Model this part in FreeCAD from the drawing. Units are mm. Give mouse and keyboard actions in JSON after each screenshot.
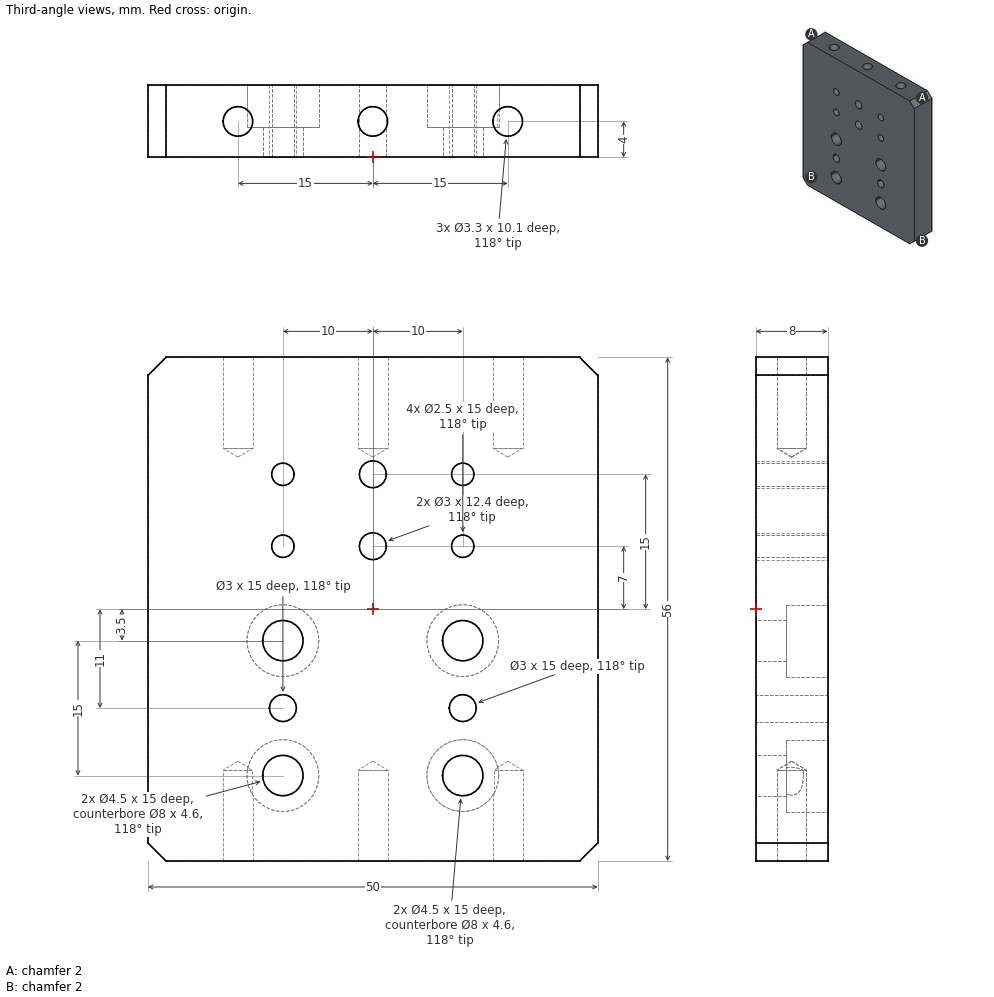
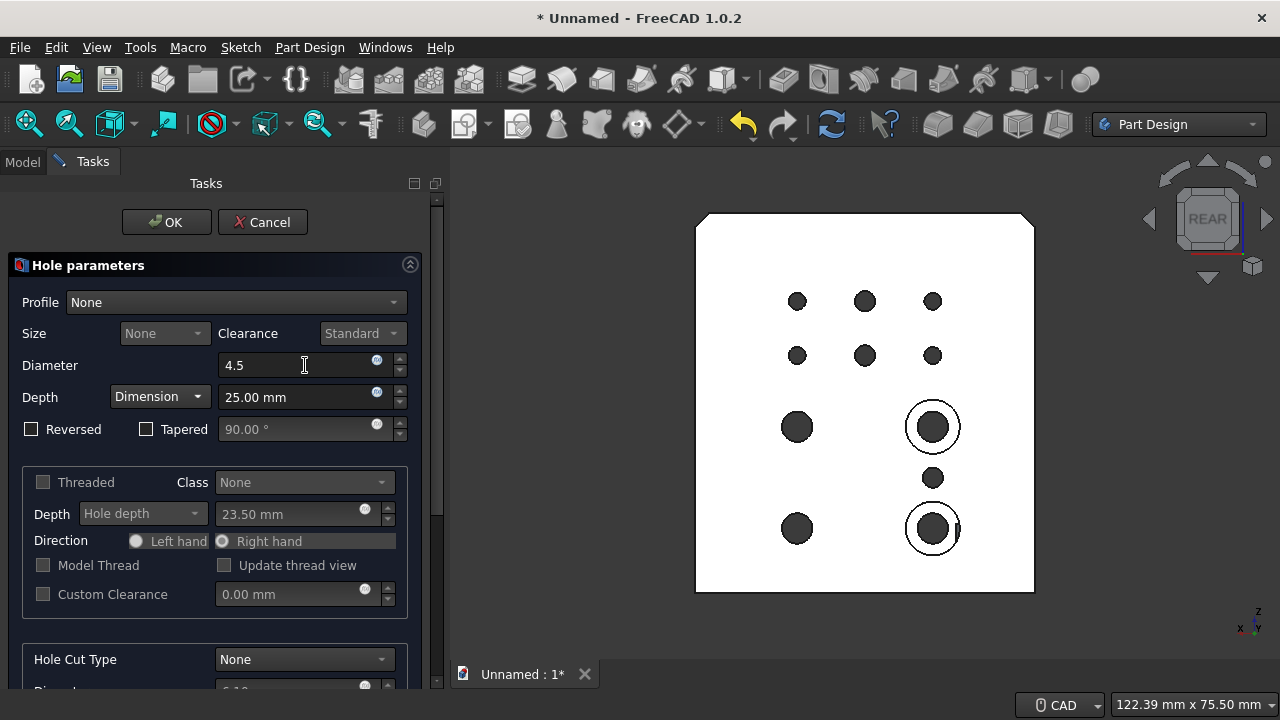
{"action": "triple_click", "coordinate": [305, 397]}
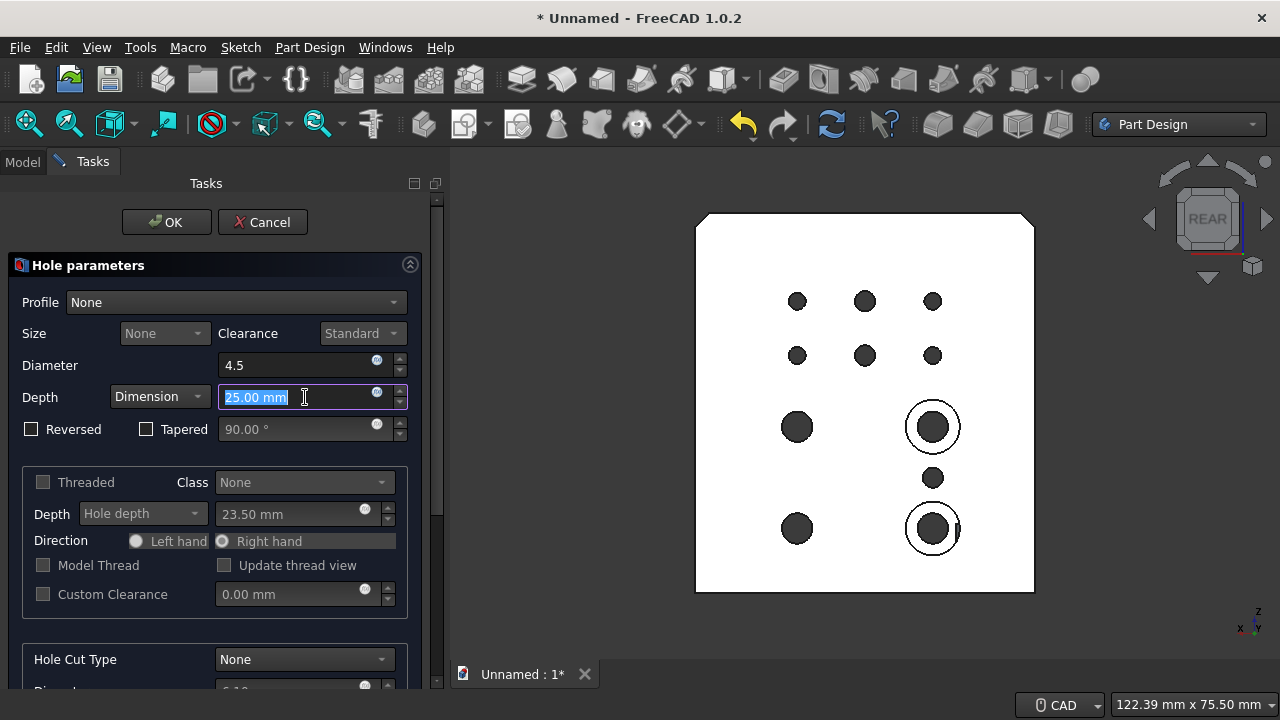
{"action": "type", "text": "15"}
{"action": "key", "text": "Tab"}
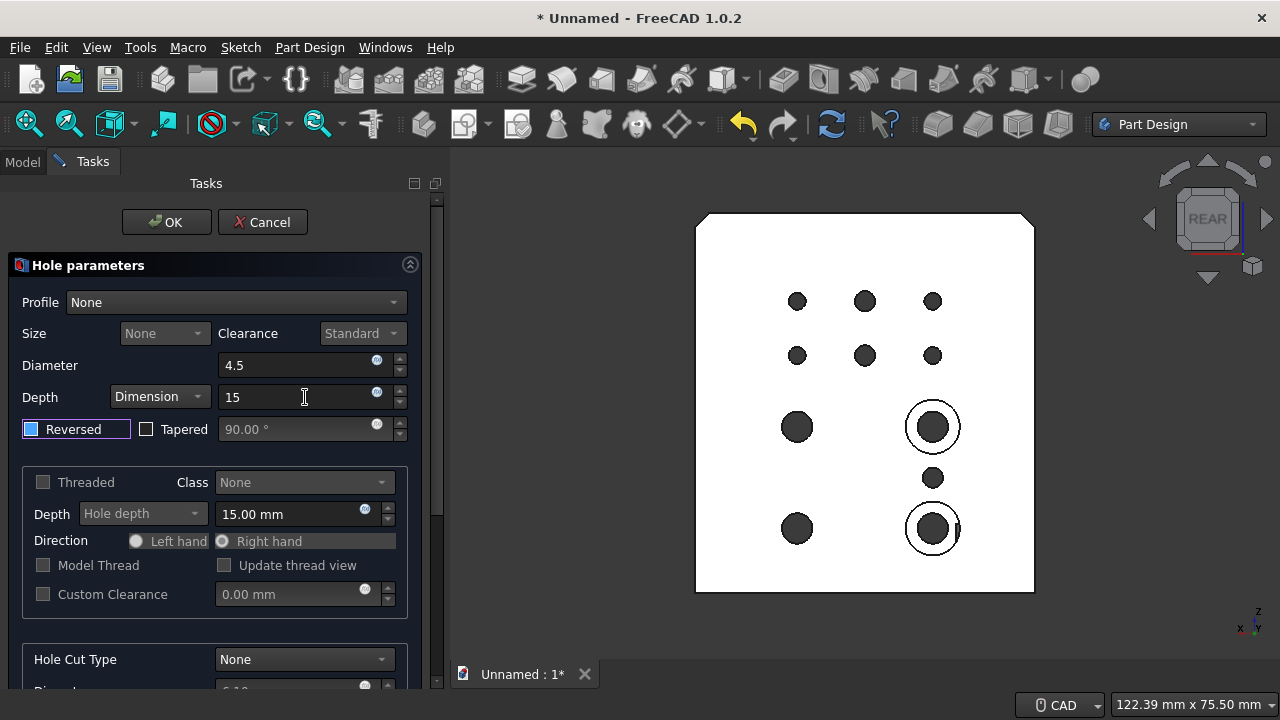
{"action": "left_click", "coordinate": [306, 660]}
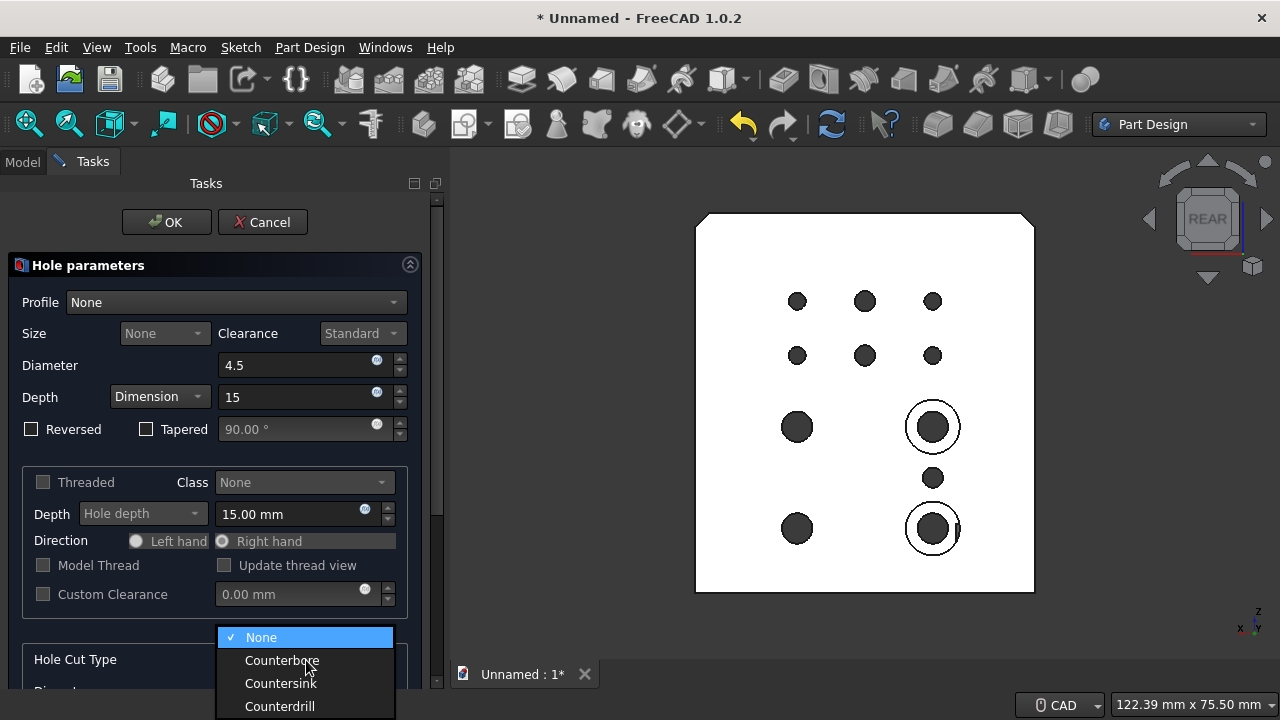
{"action": "left_click", "coordinate": [304, 660]}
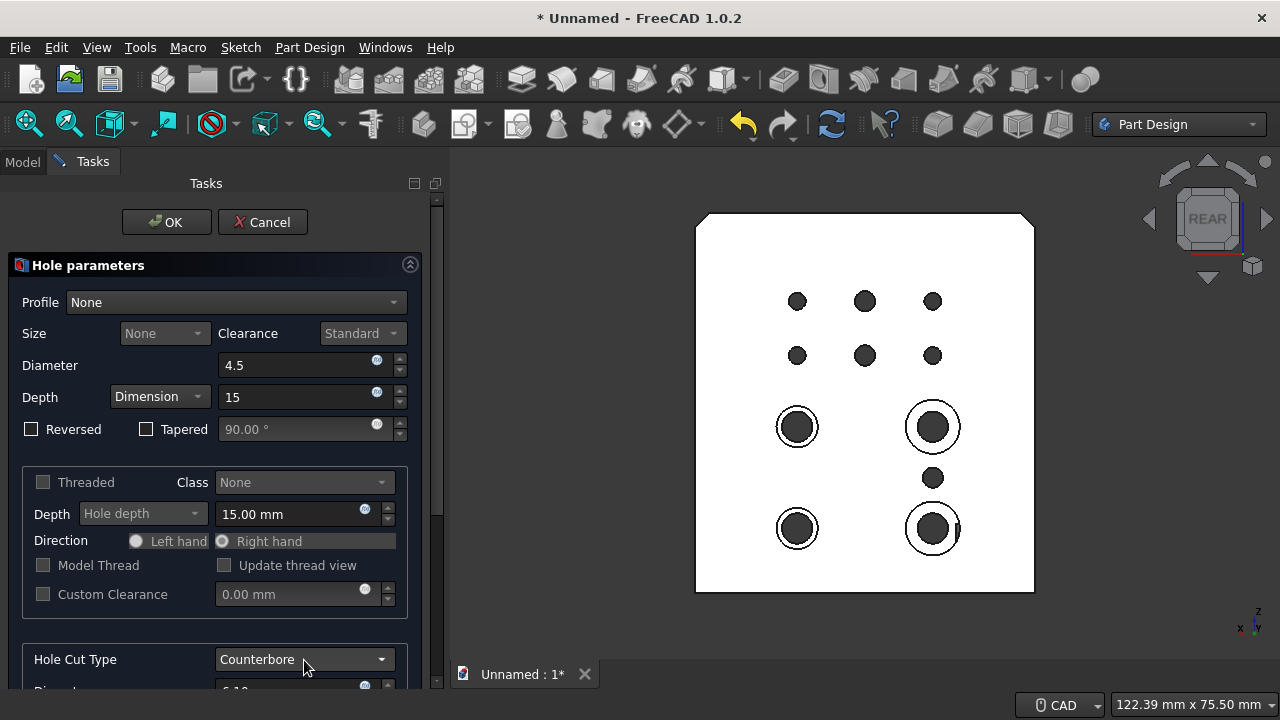
{"action": "scroll", "coordinate": [437, 440], "scroll_direction": "down", "scroll_amount": 2}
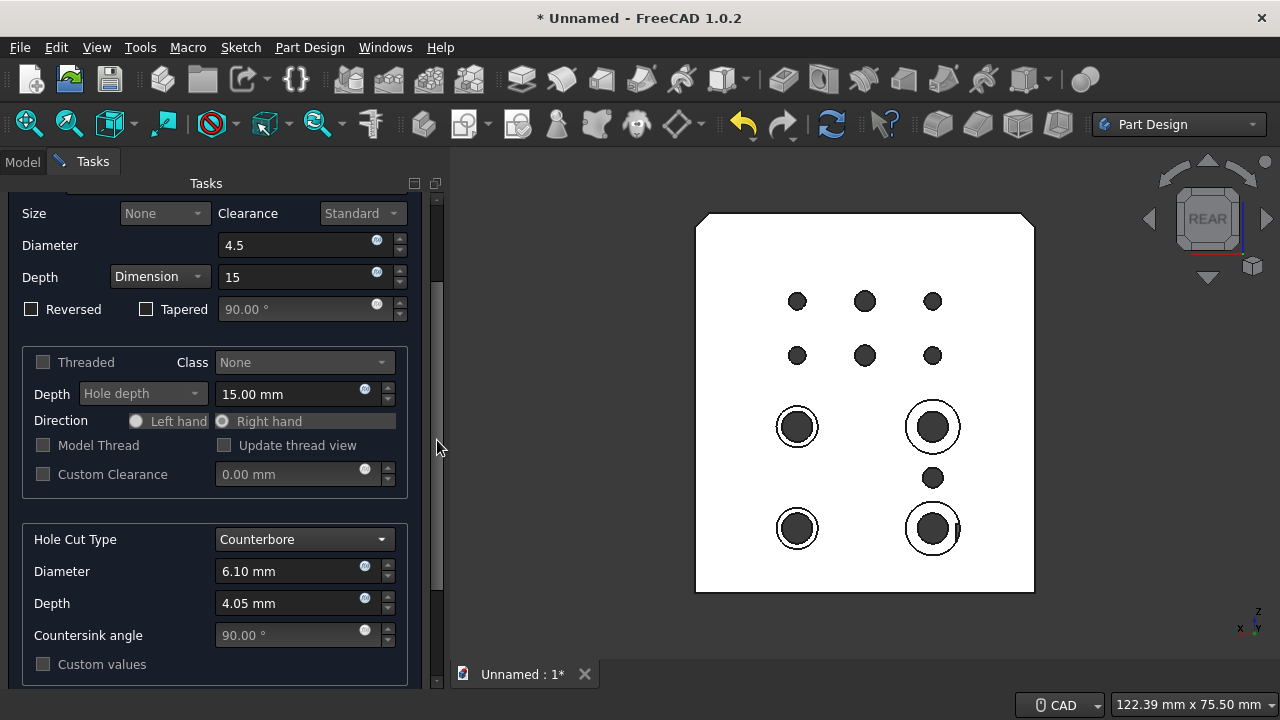
{"action": "triple_click", "coordinate": [298, 571]}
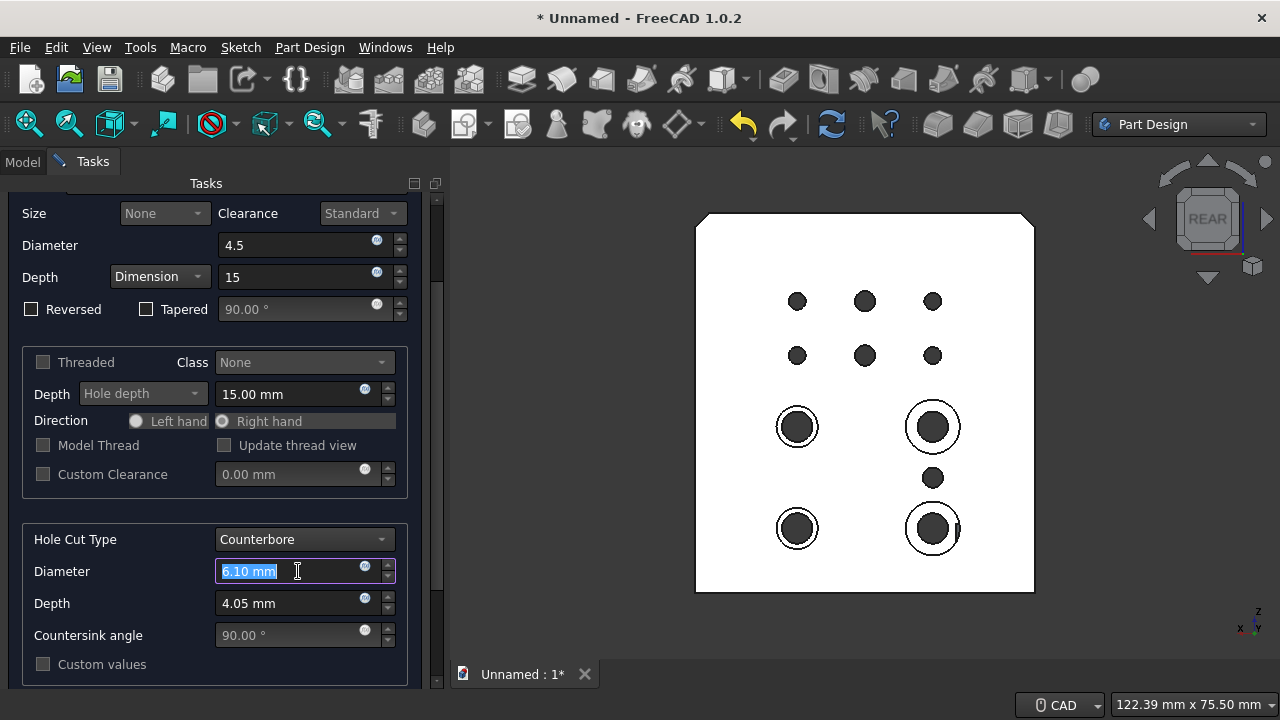
{"action": "type", "text": "8"}
{"action": "key", "text": "Tab"}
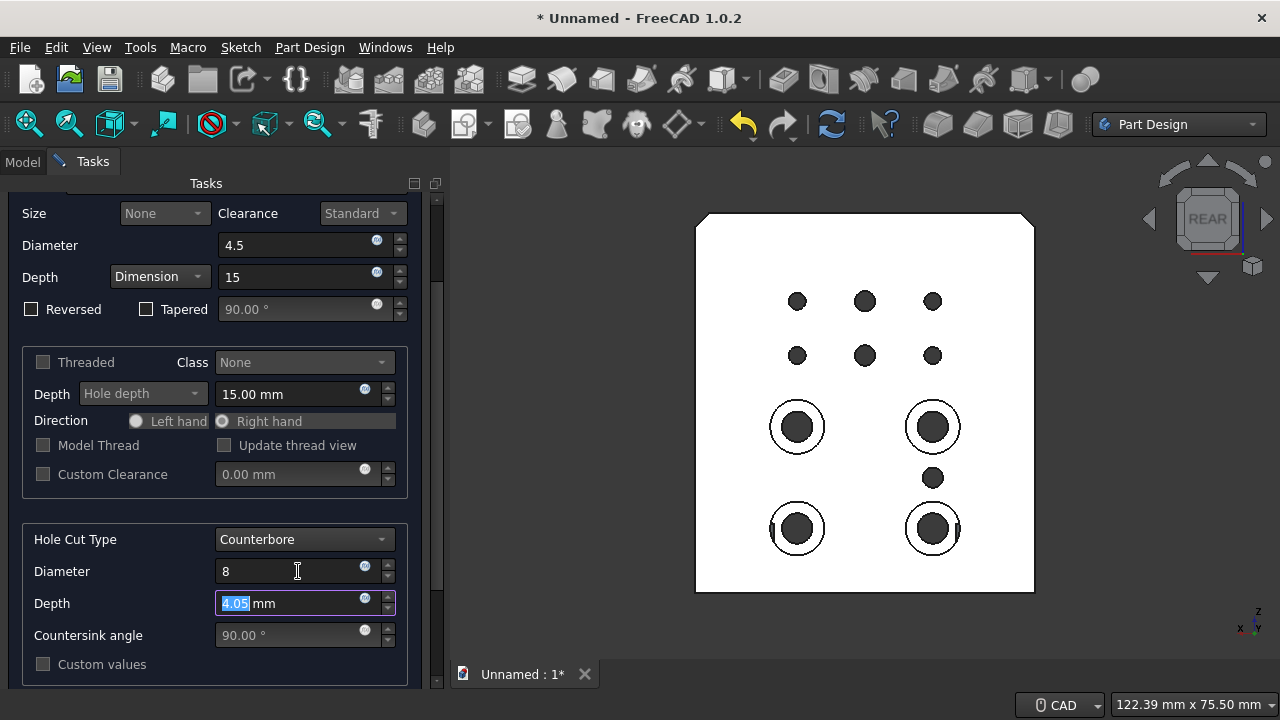
{"action": "type", "text": "4.6"}
{"action": "key", "text": "Tab"}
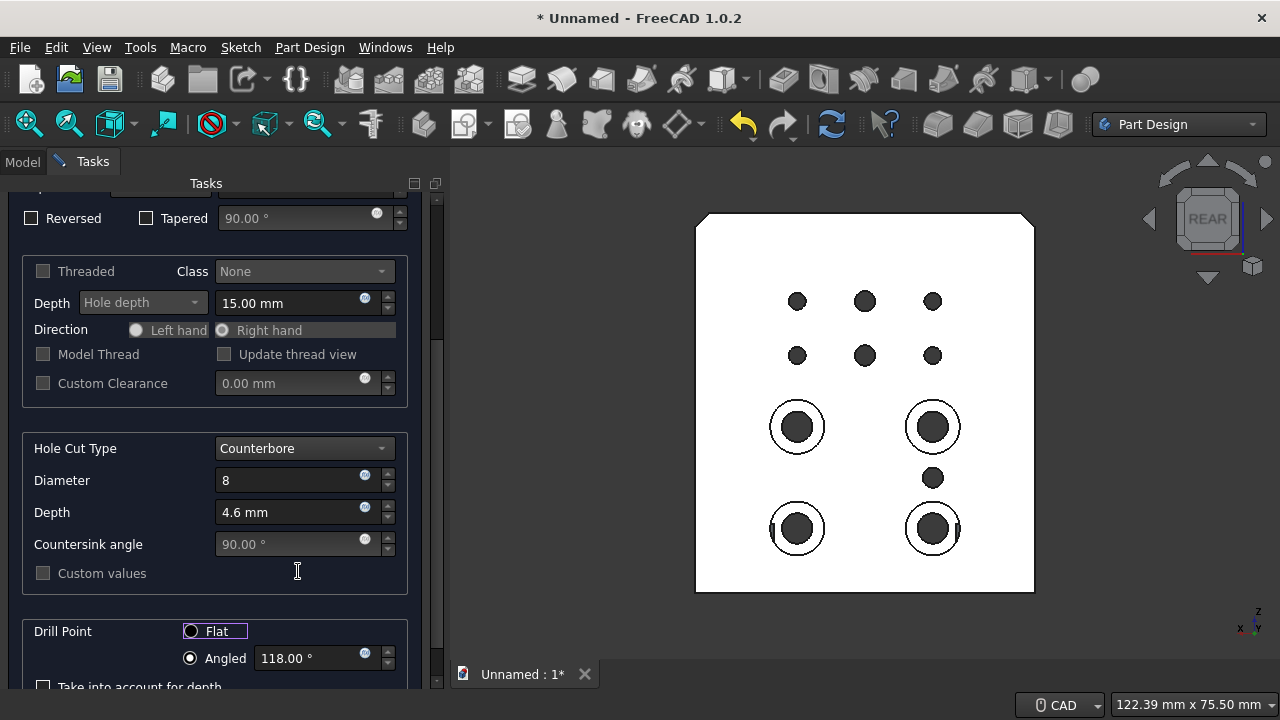
{"action": "scroll", "coordinate": [437, 440], "scroll_direction": "up", "scroll_amount": 5}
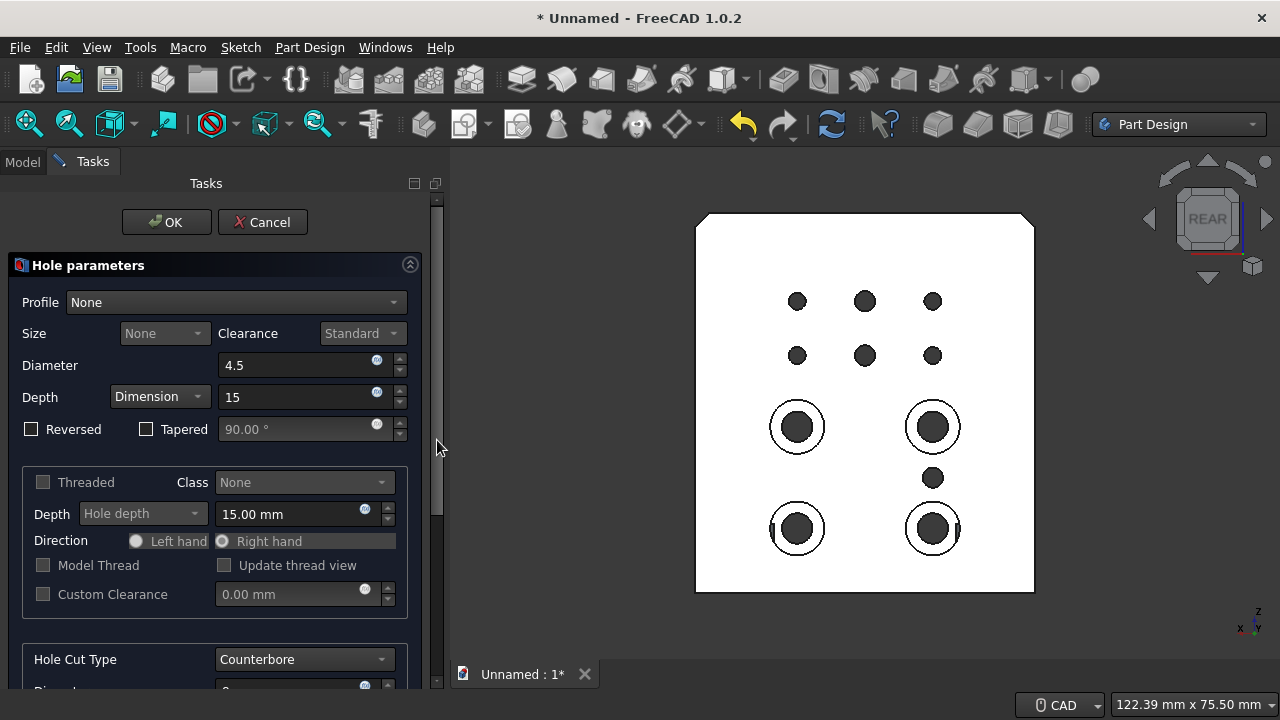
{"action": "left_click", "coordinate": [167, 222]}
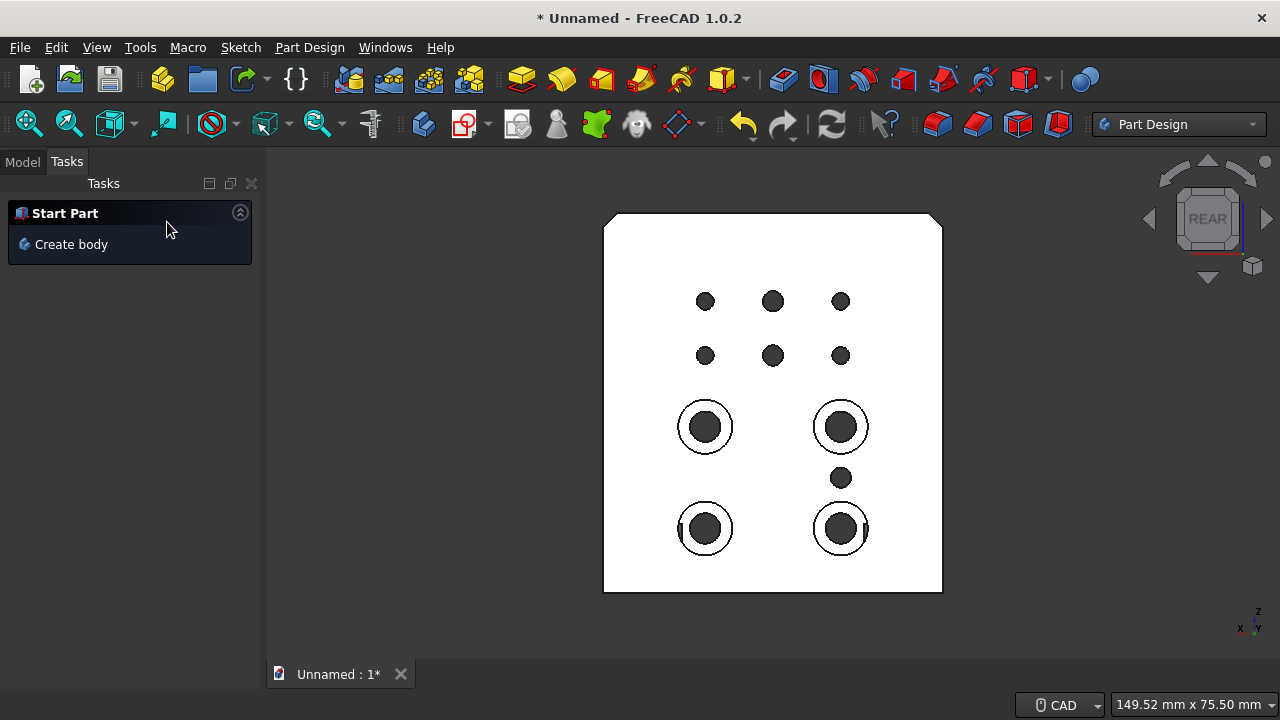
{"action": "left_click", "coordinate": [773, 456]}